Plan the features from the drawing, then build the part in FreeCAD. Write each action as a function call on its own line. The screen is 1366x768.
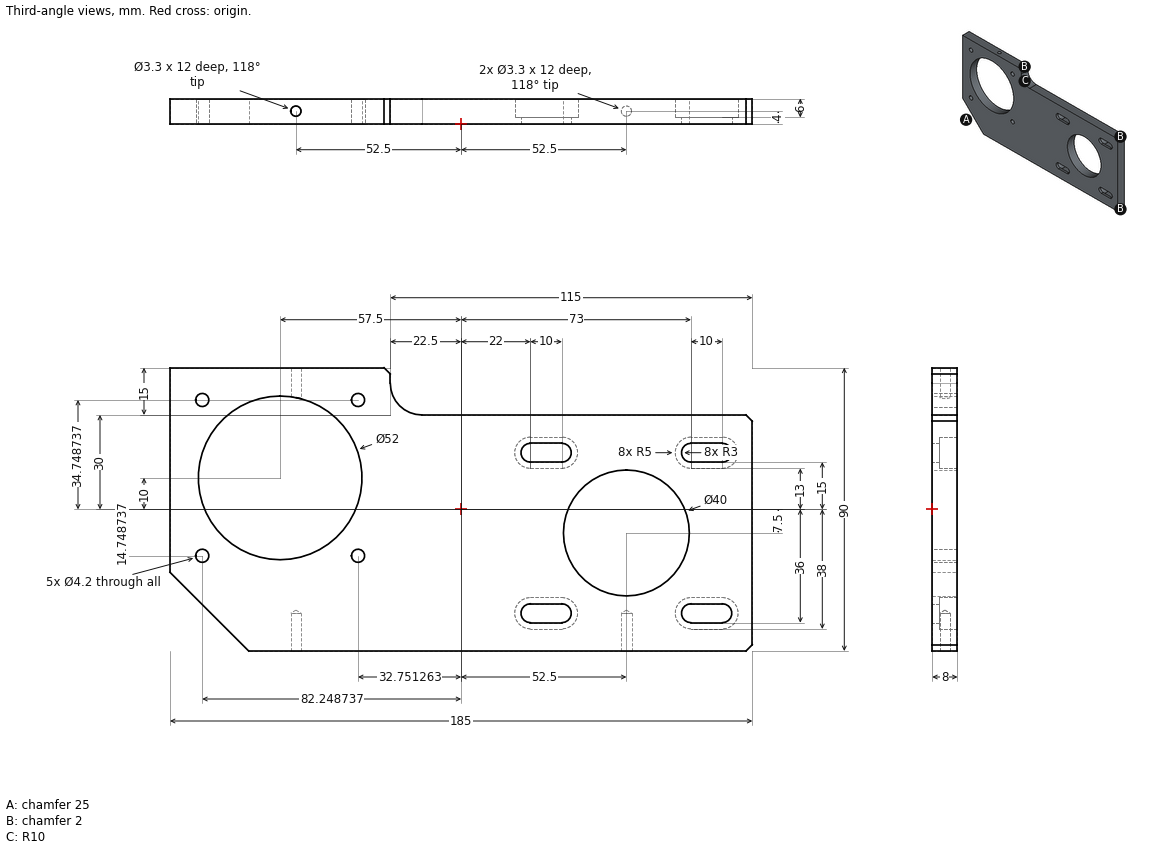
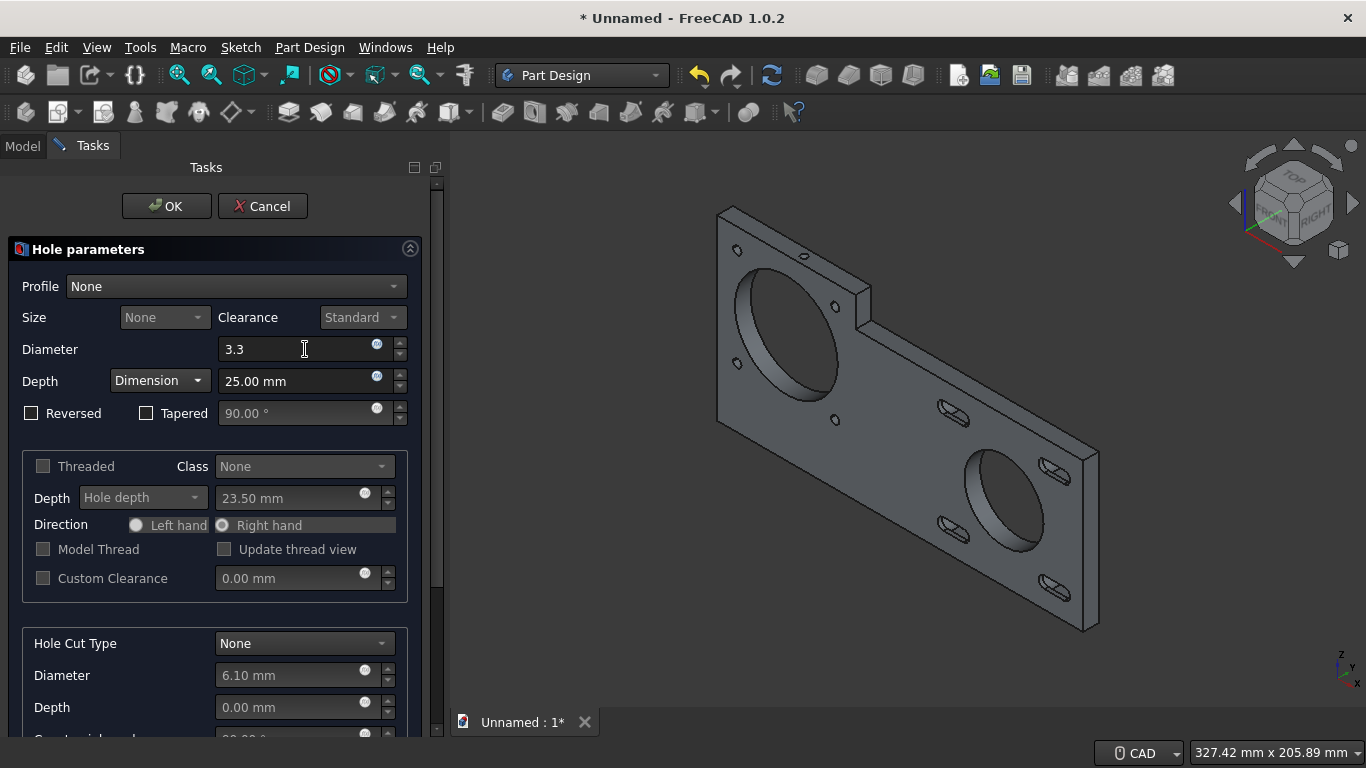
triple_click(305, 381)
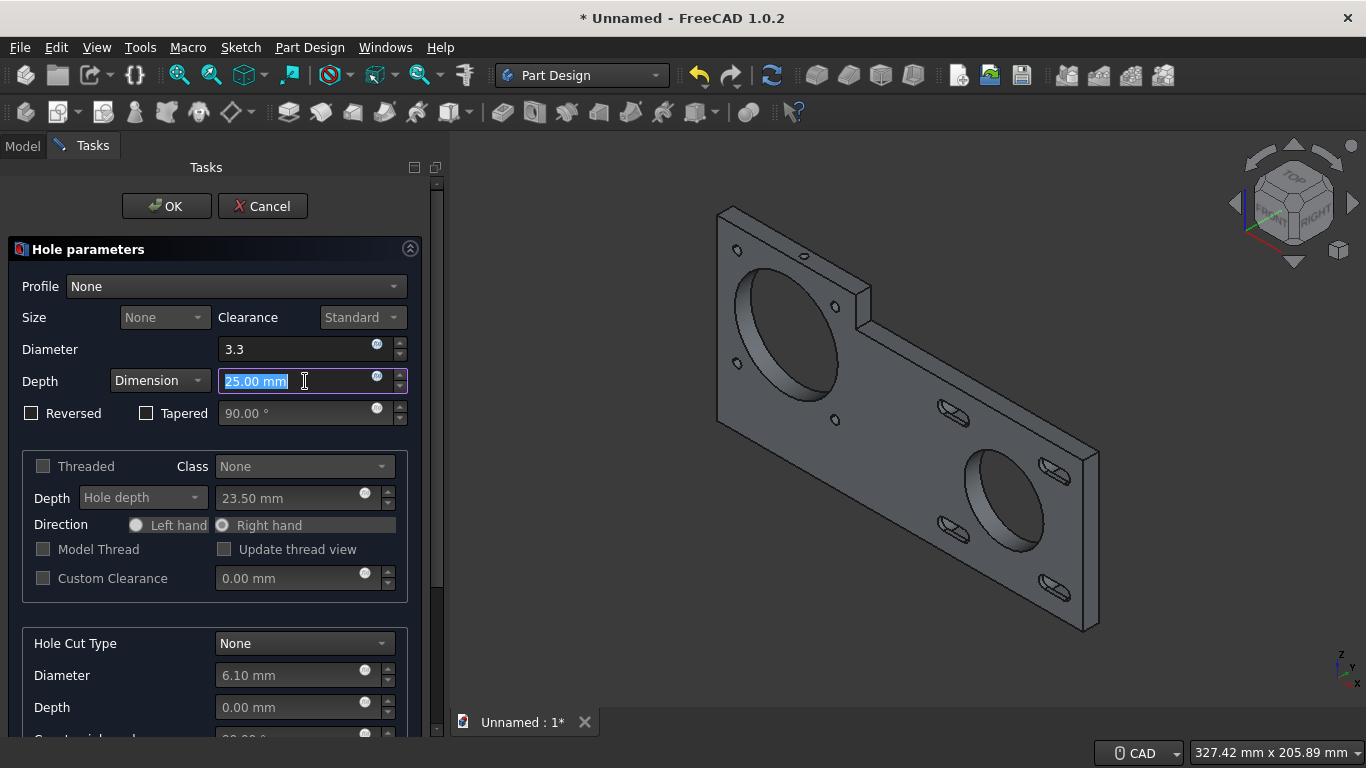
text(12)
key(Tab)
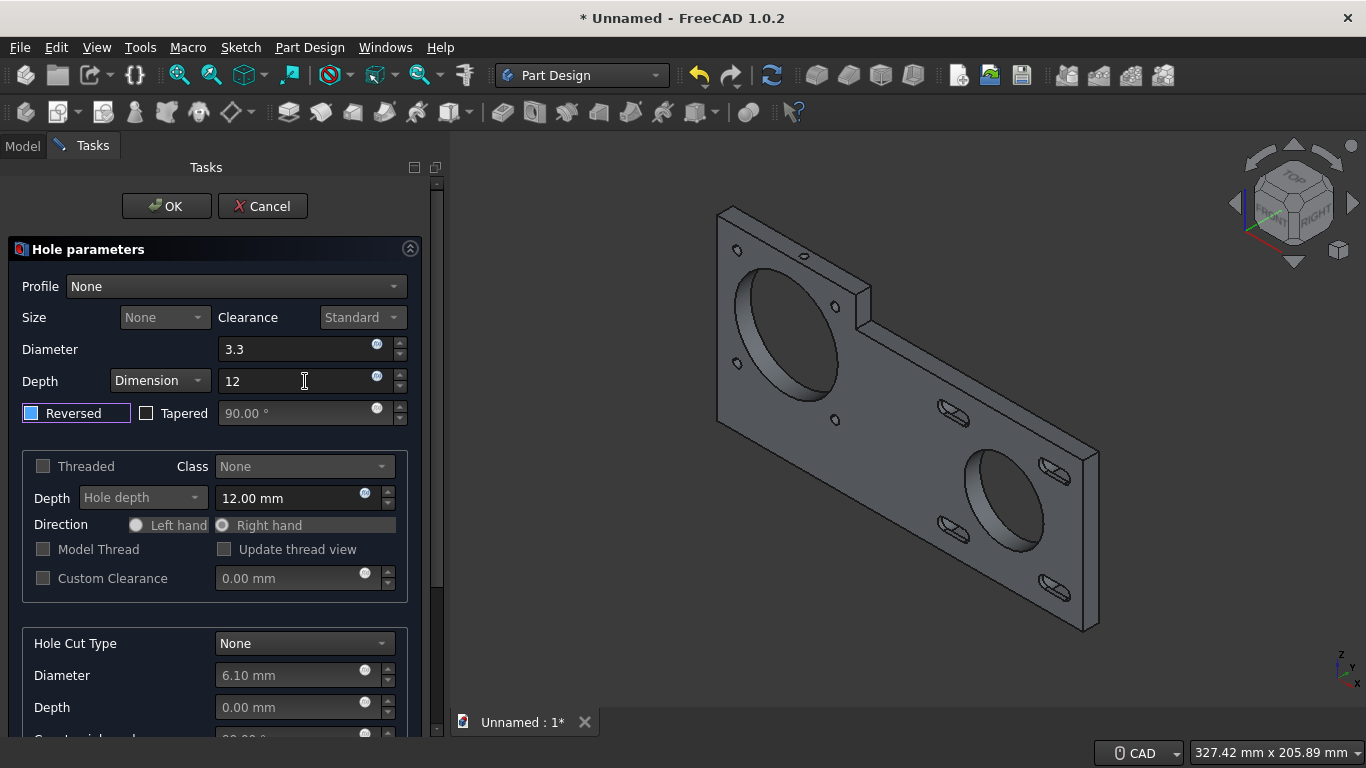
click(167, 206)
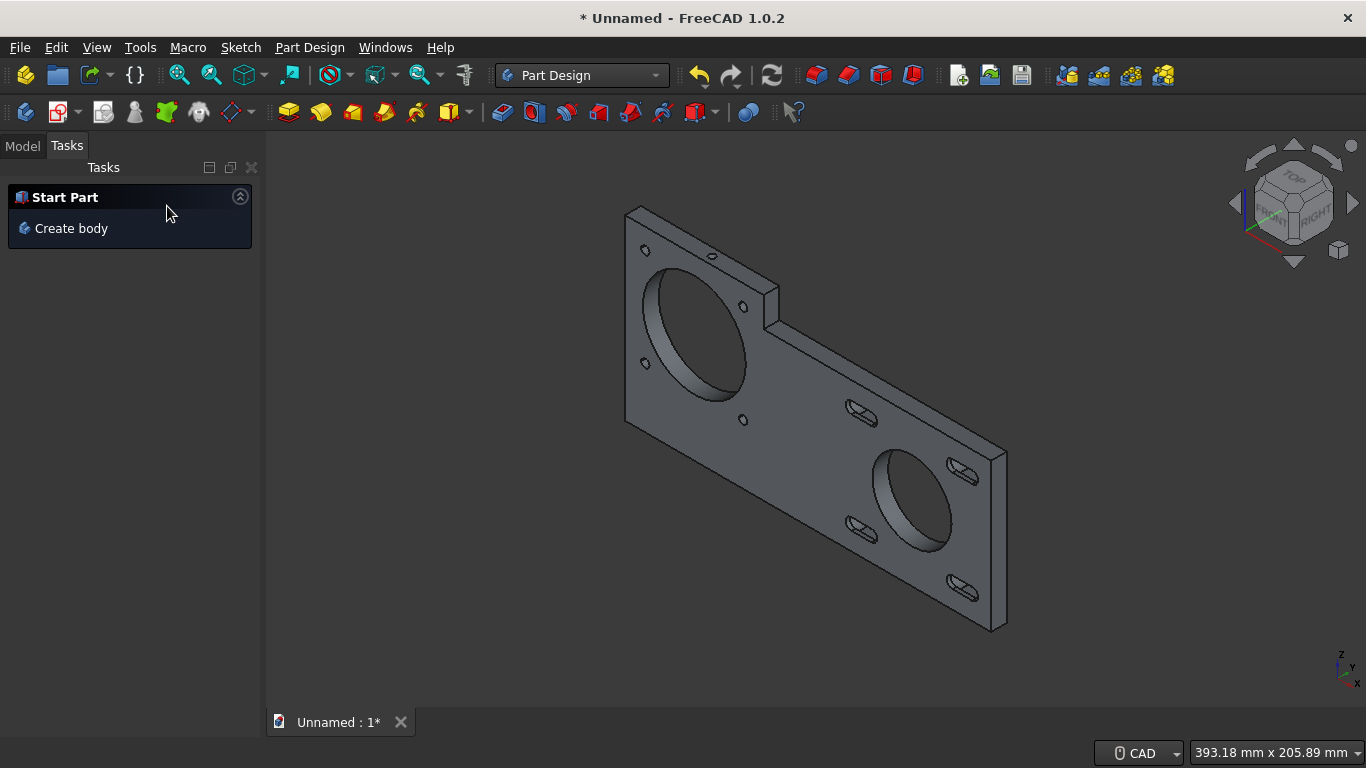
key(2)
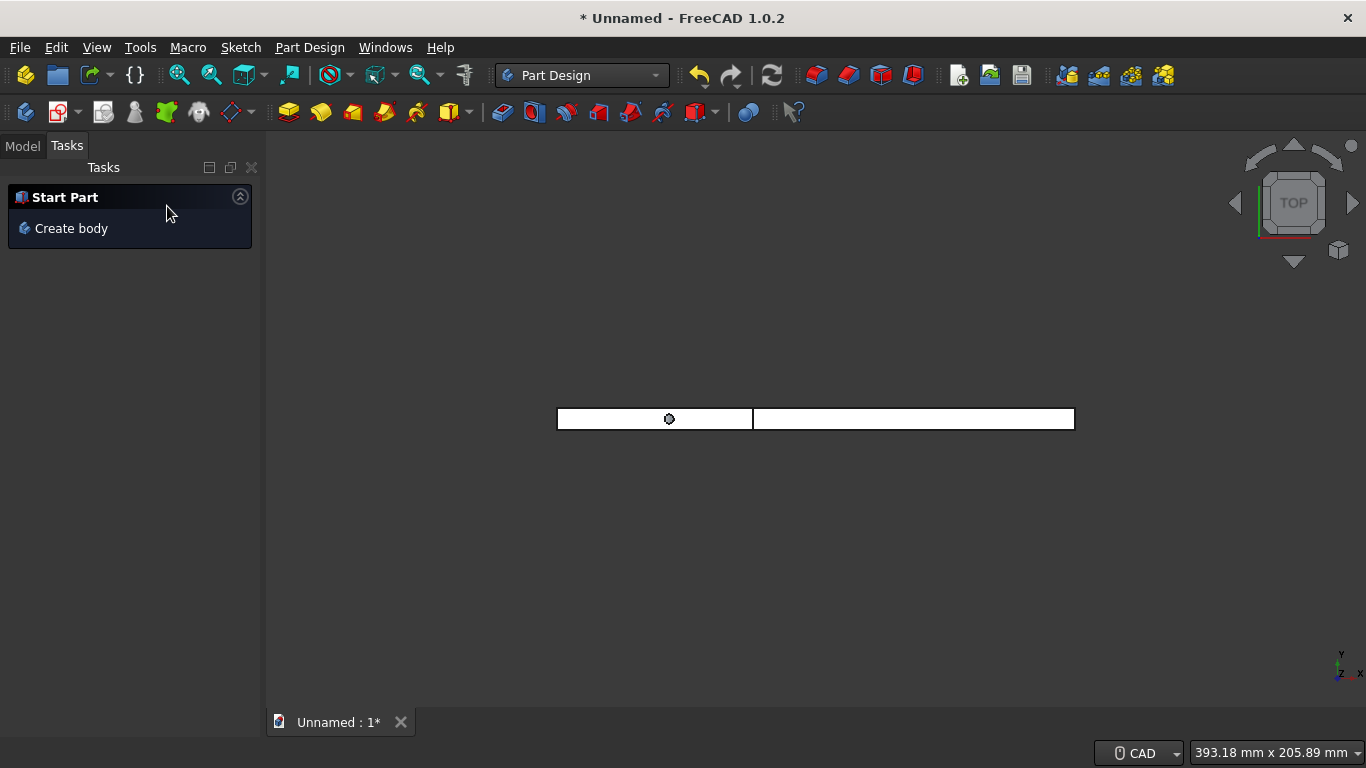
key(0)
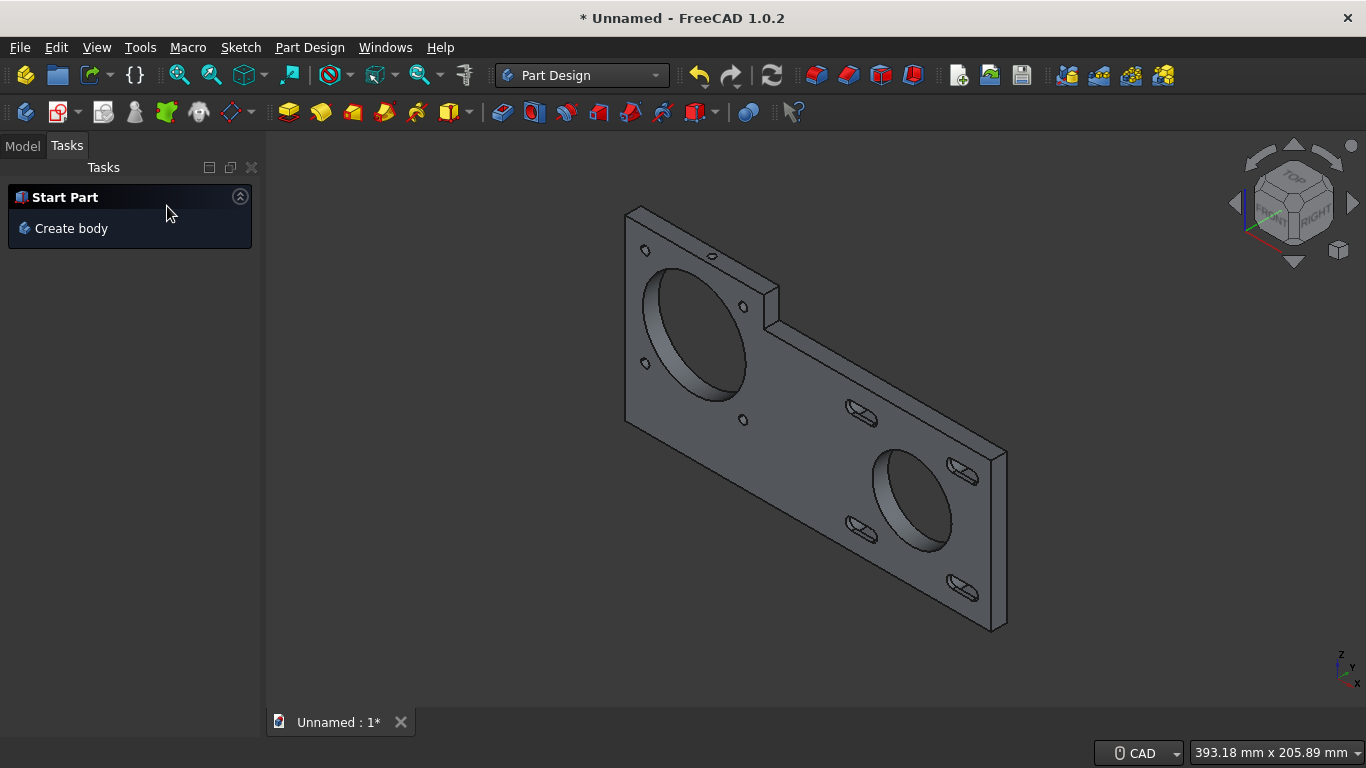
key(1)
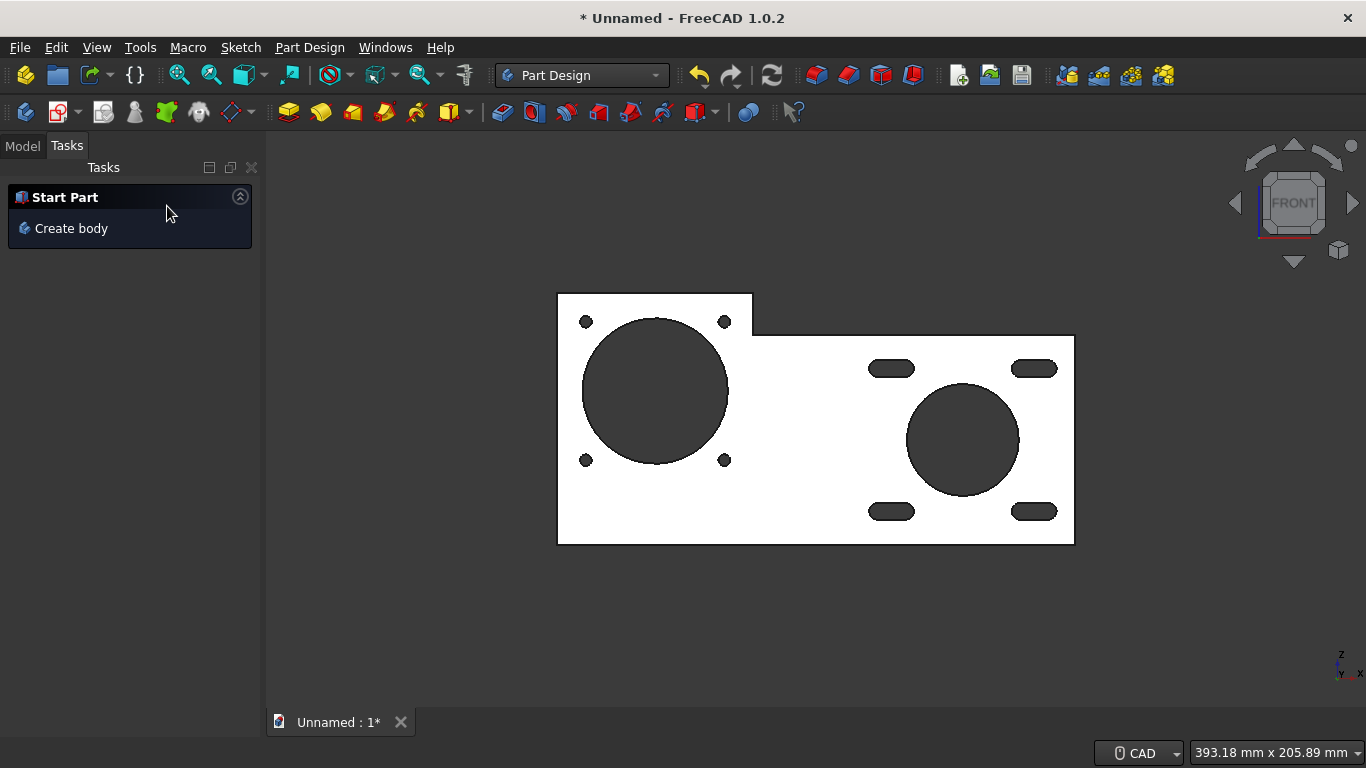
key(3)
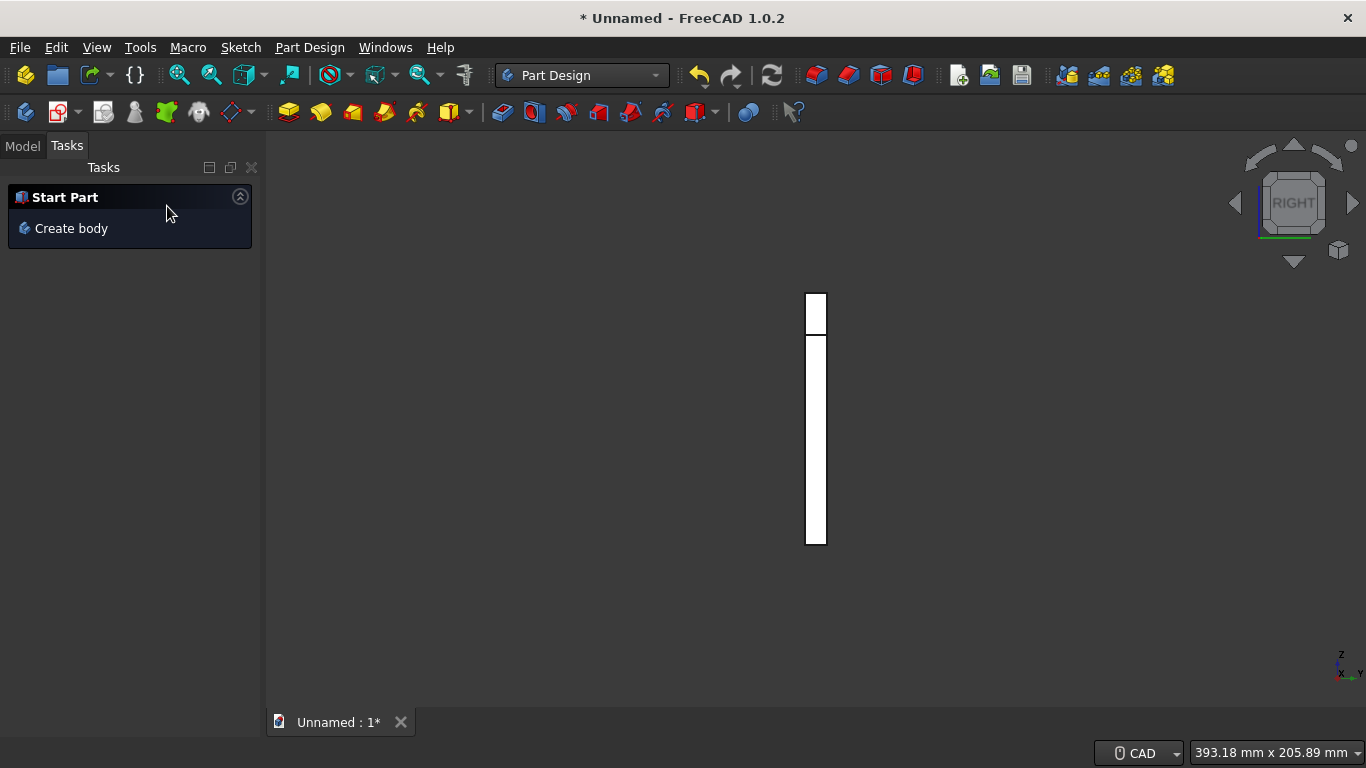
click(180, 76)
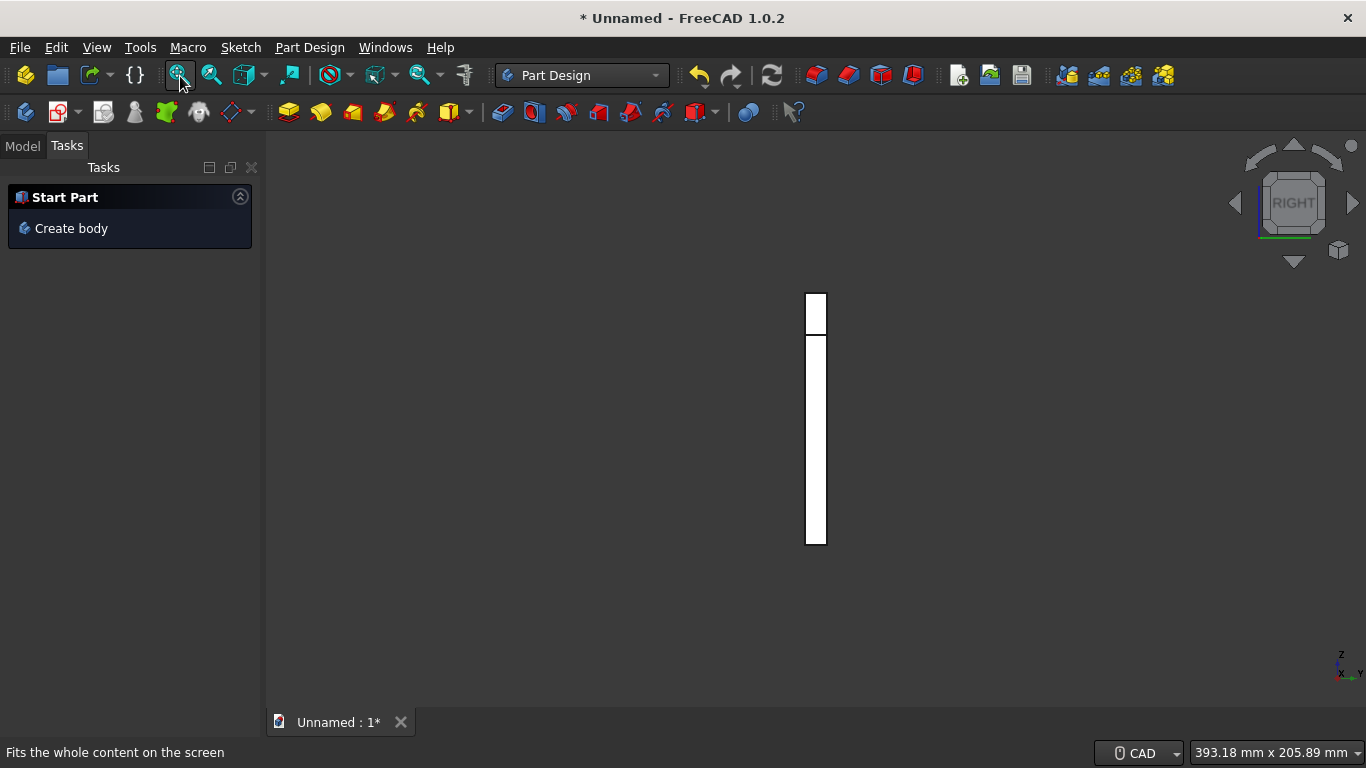
key(5)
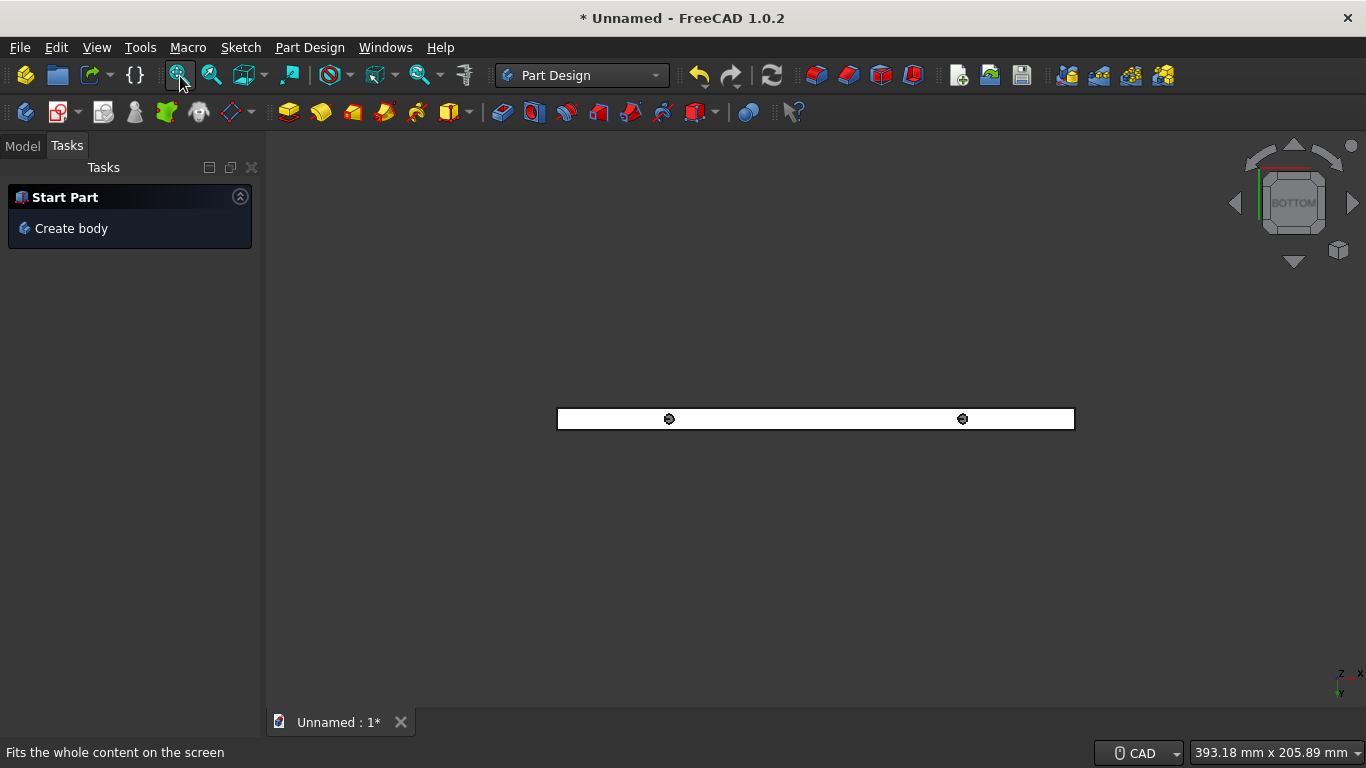
click(557, 418)